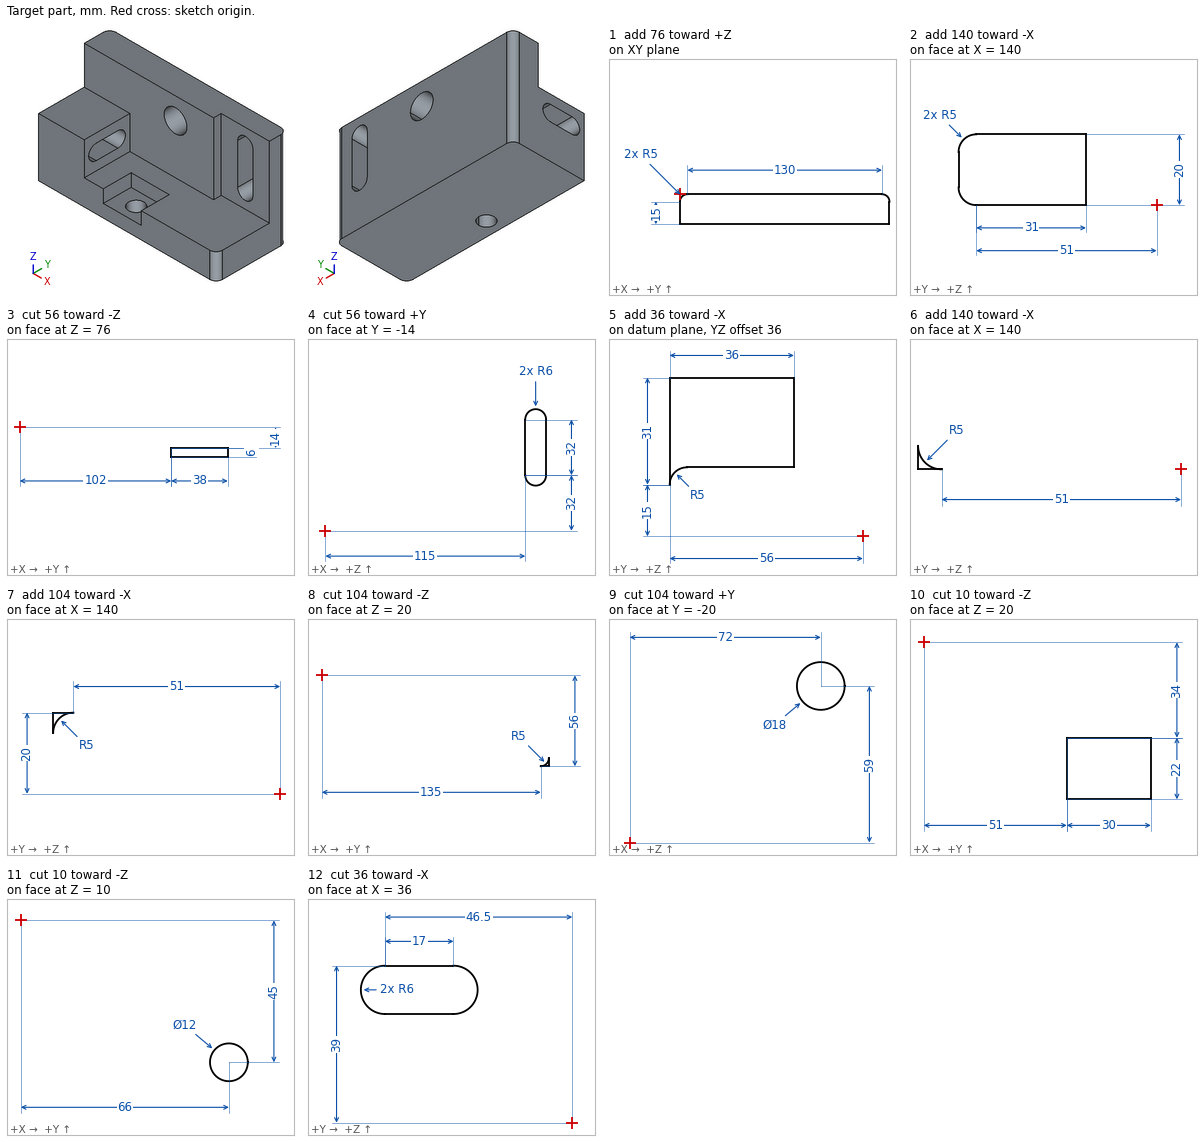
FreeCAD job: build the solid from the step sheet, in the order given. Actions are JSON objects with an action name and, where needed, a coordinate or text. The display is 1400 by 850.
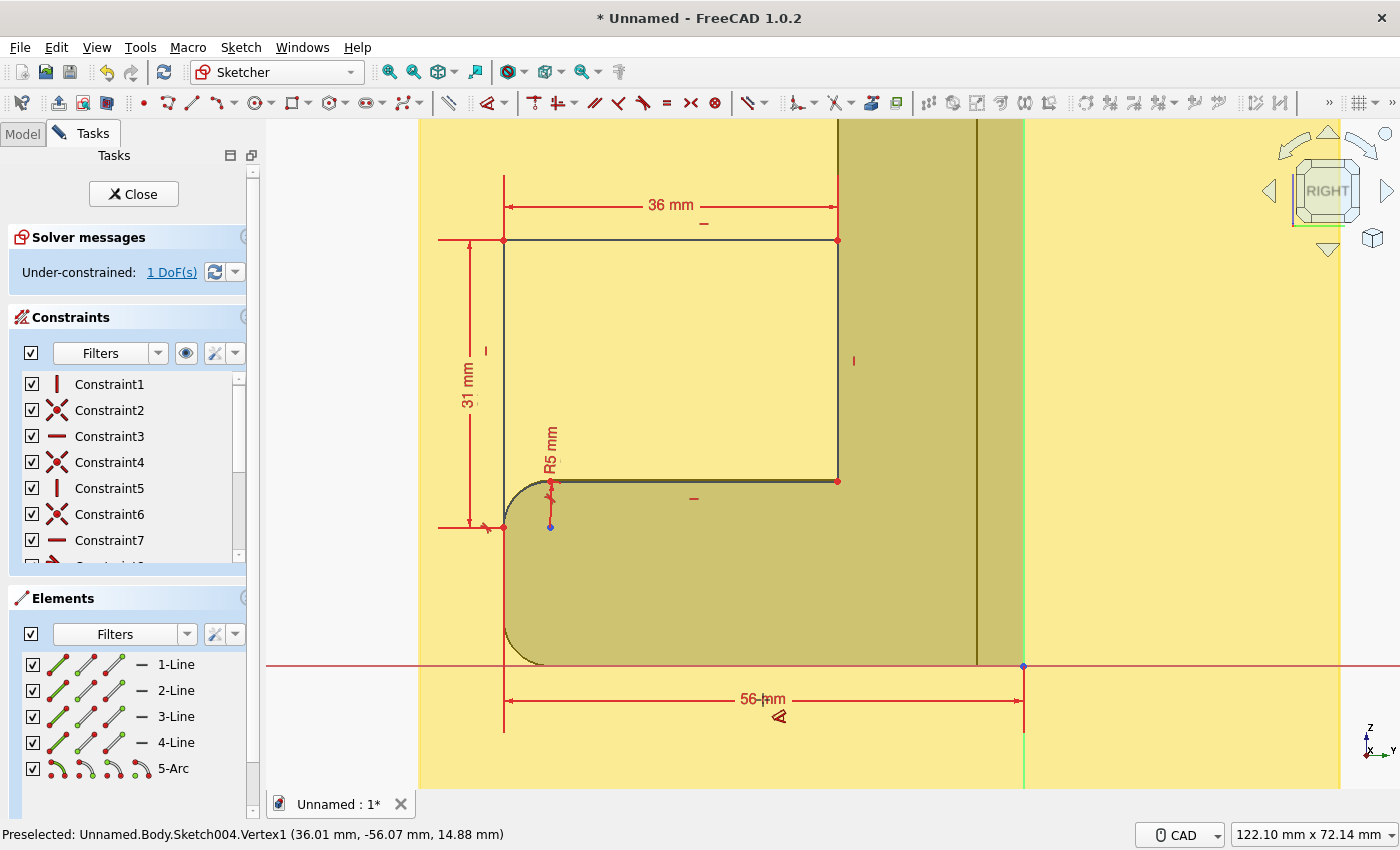
{"action": "left_click", "coordinate": [504, 528]}
{"action": "left_click", "coordinate": [1058, 597]}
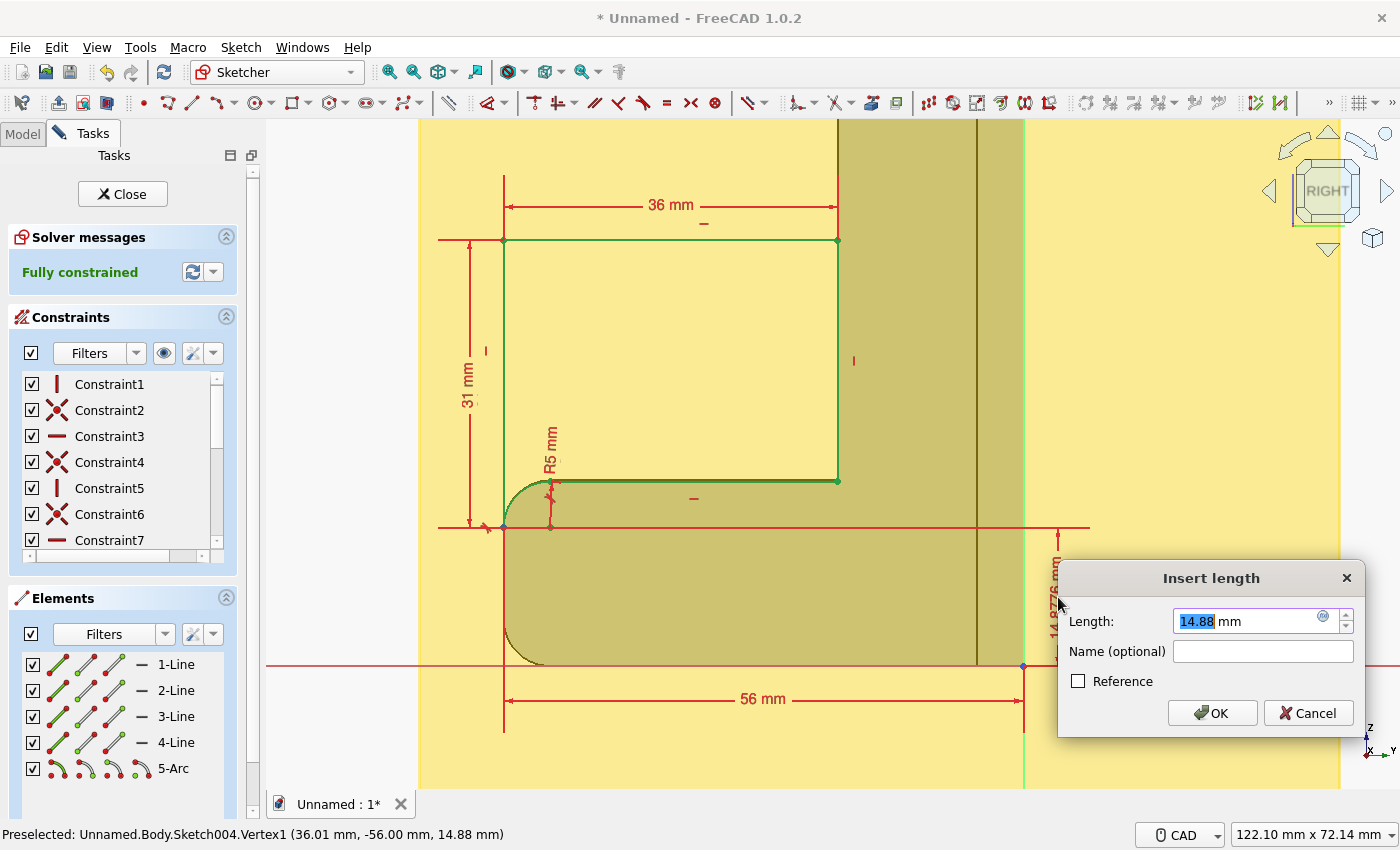
{"action": "type", "text": "15"}
{"action": "key", "text": "Return"}
{"action": "key", "text": "Escape"}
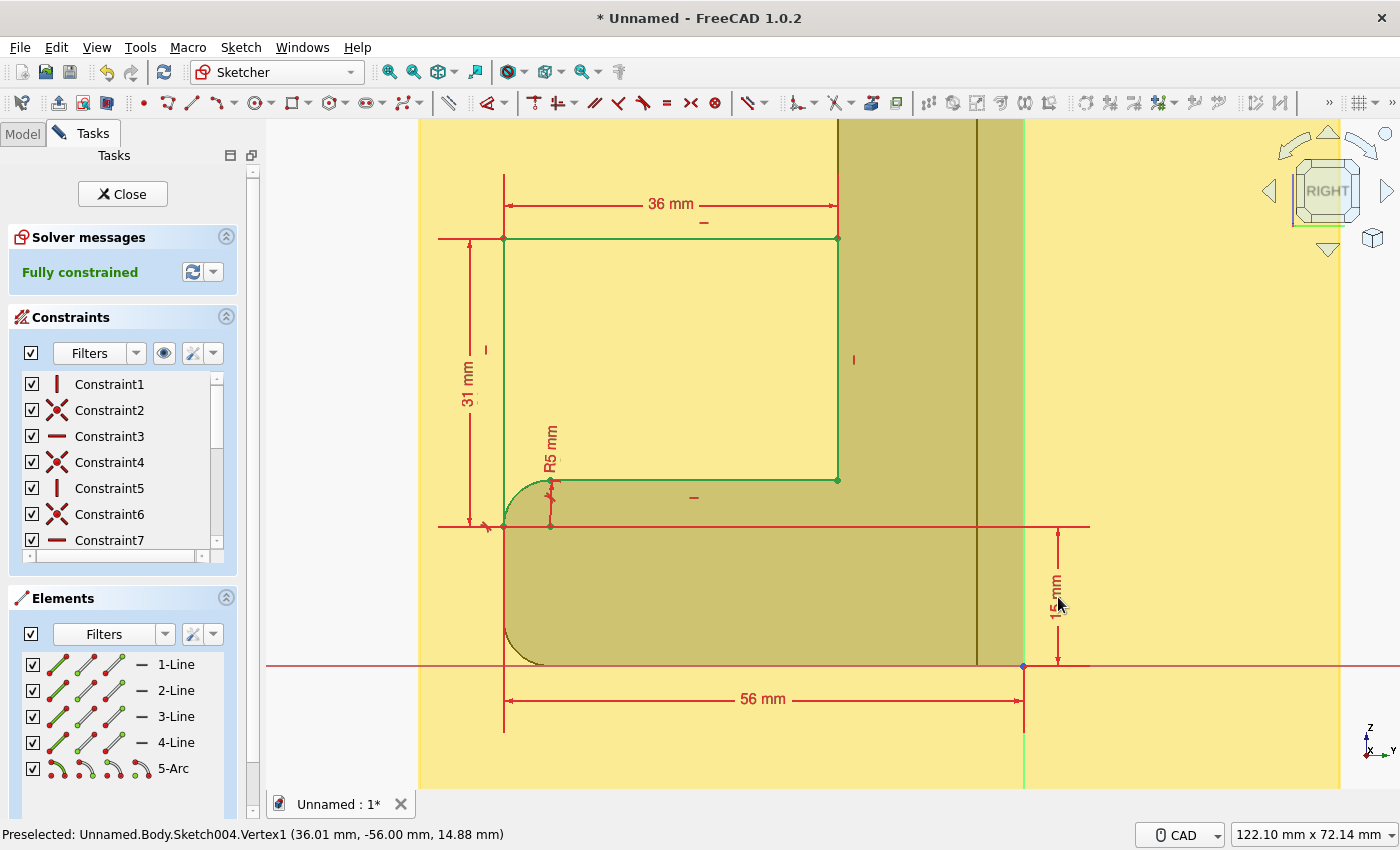
{"action": "left_click", "coordinate": [123, 194]}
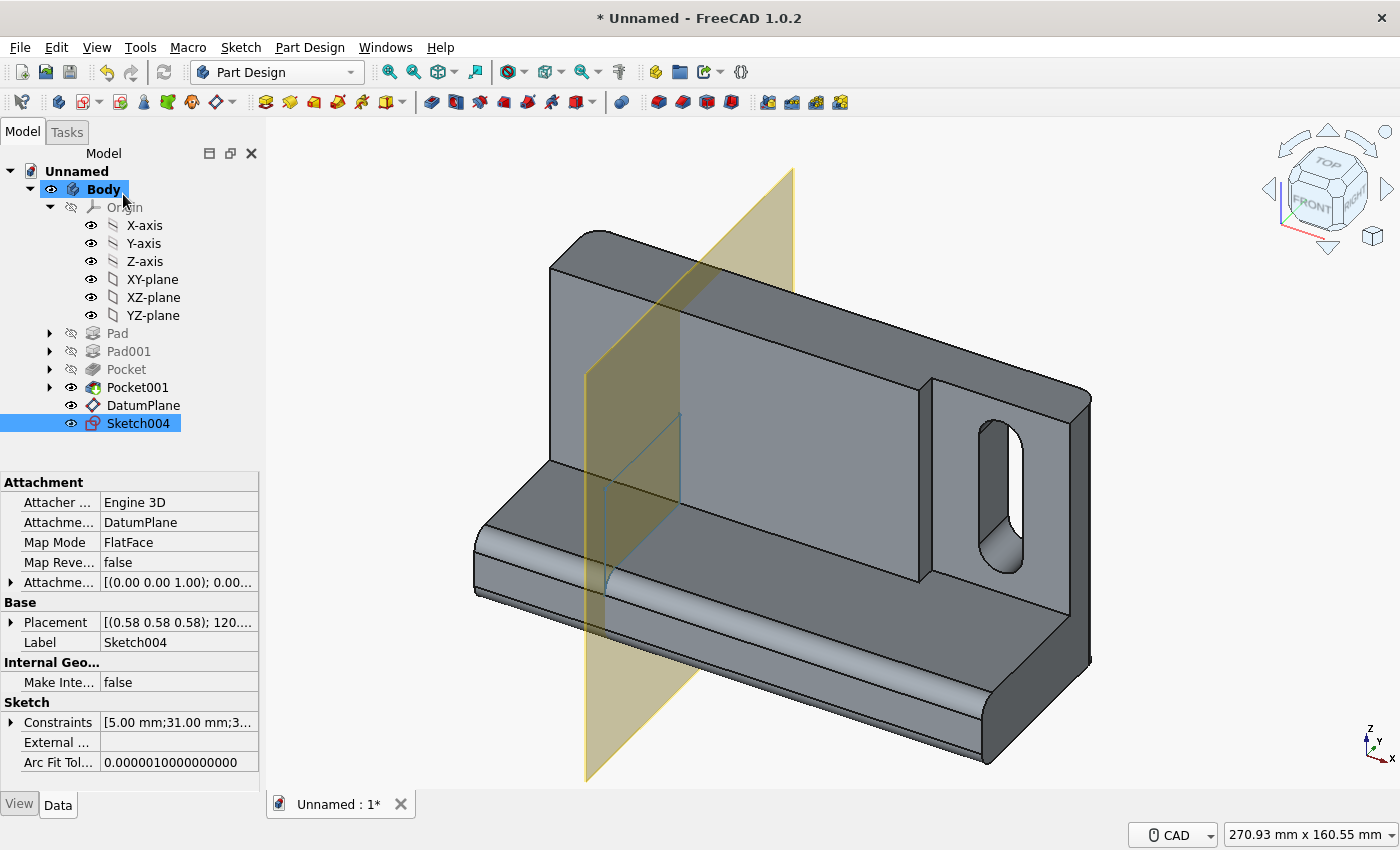
{"action": "left_click", "coordinate": [266, 102]}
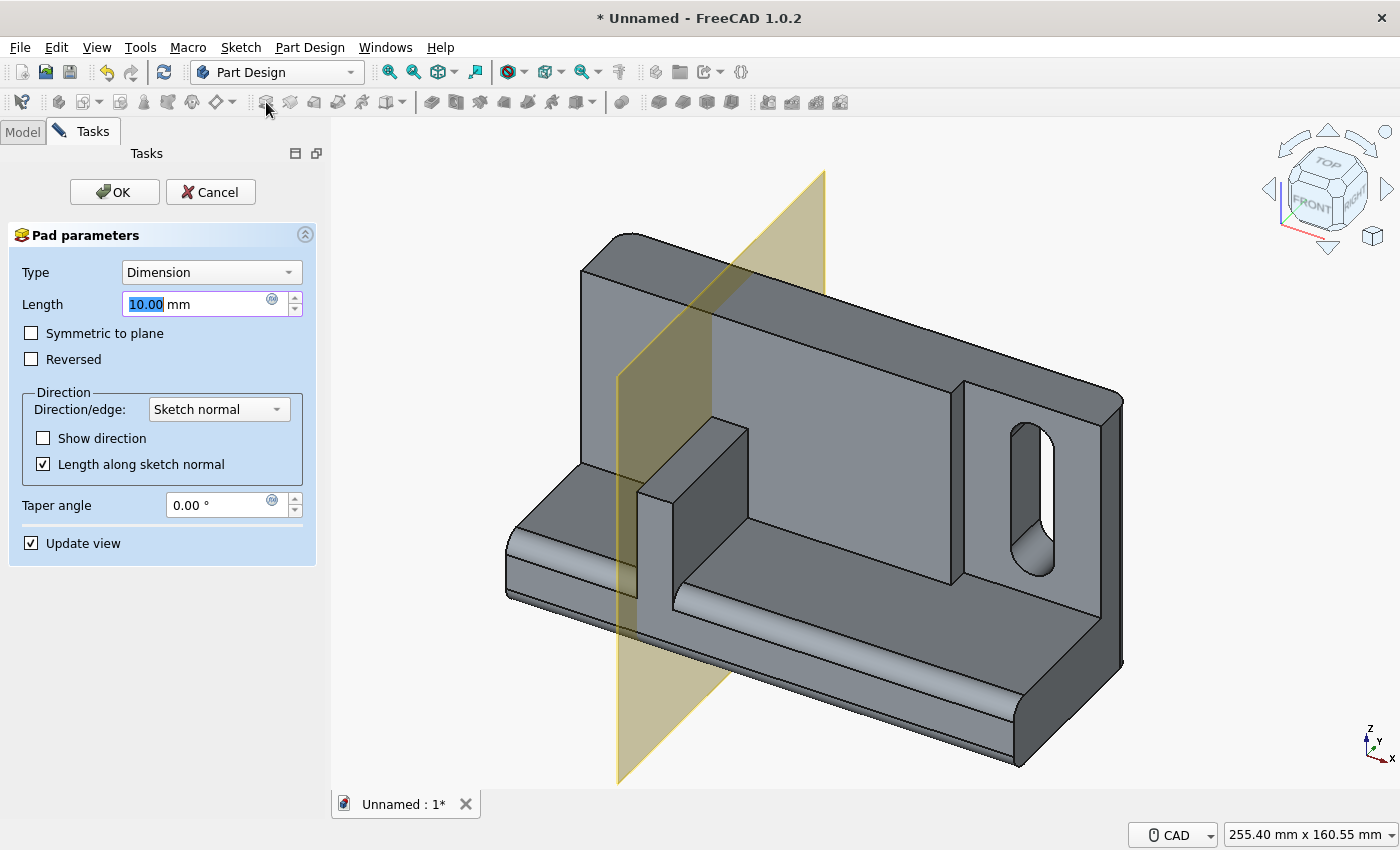
{"action": "type", "text": "36"}
{"action": "key", "text": "Tab"}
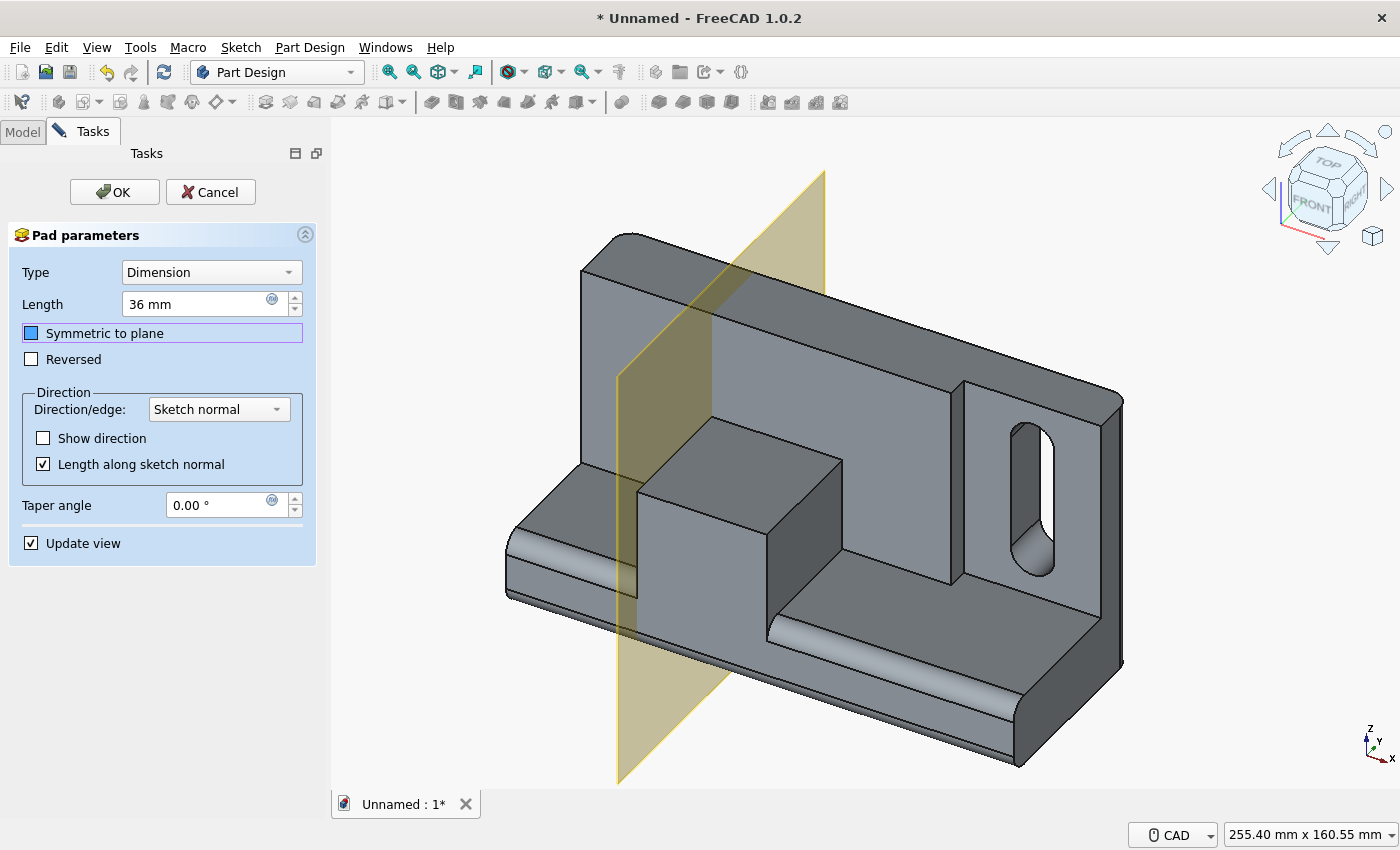
{"action": "left_click", "coordinate": [30, 359]}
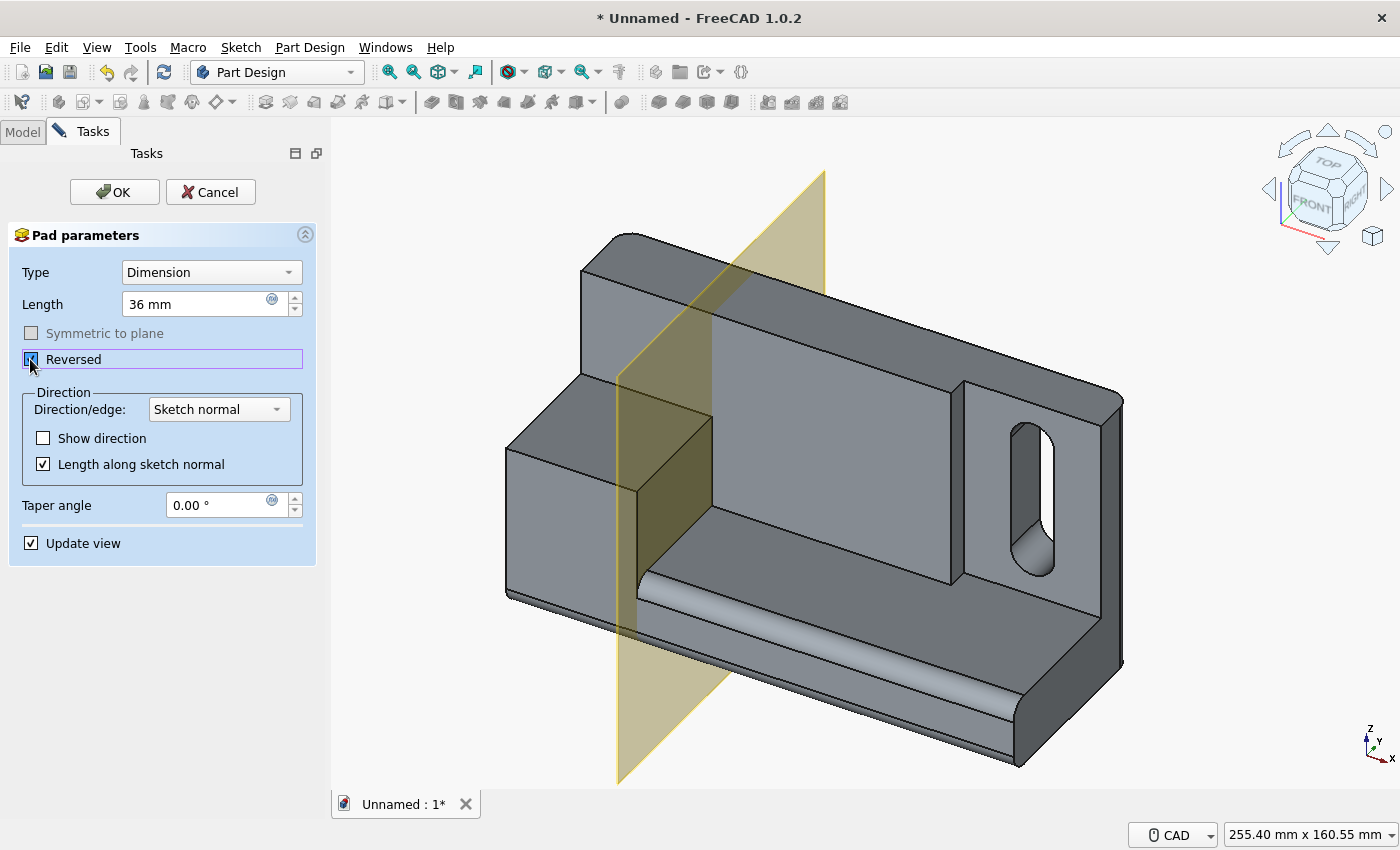
{"action": "left_click", "coordinate": [115, 192]}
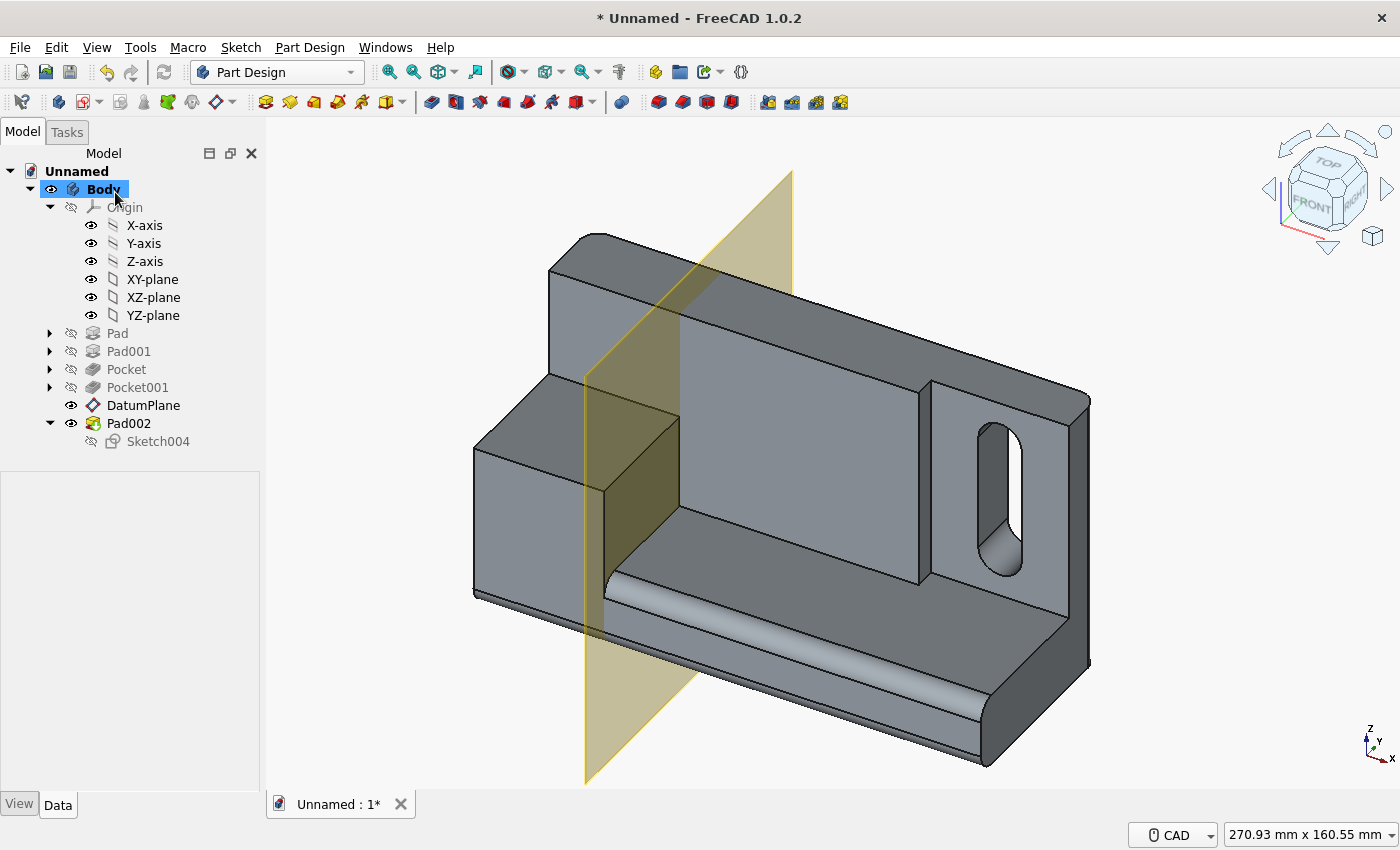
{"action": "left_click", "coordinate": [116, 405]}
{"action": "key", "text": "space"}